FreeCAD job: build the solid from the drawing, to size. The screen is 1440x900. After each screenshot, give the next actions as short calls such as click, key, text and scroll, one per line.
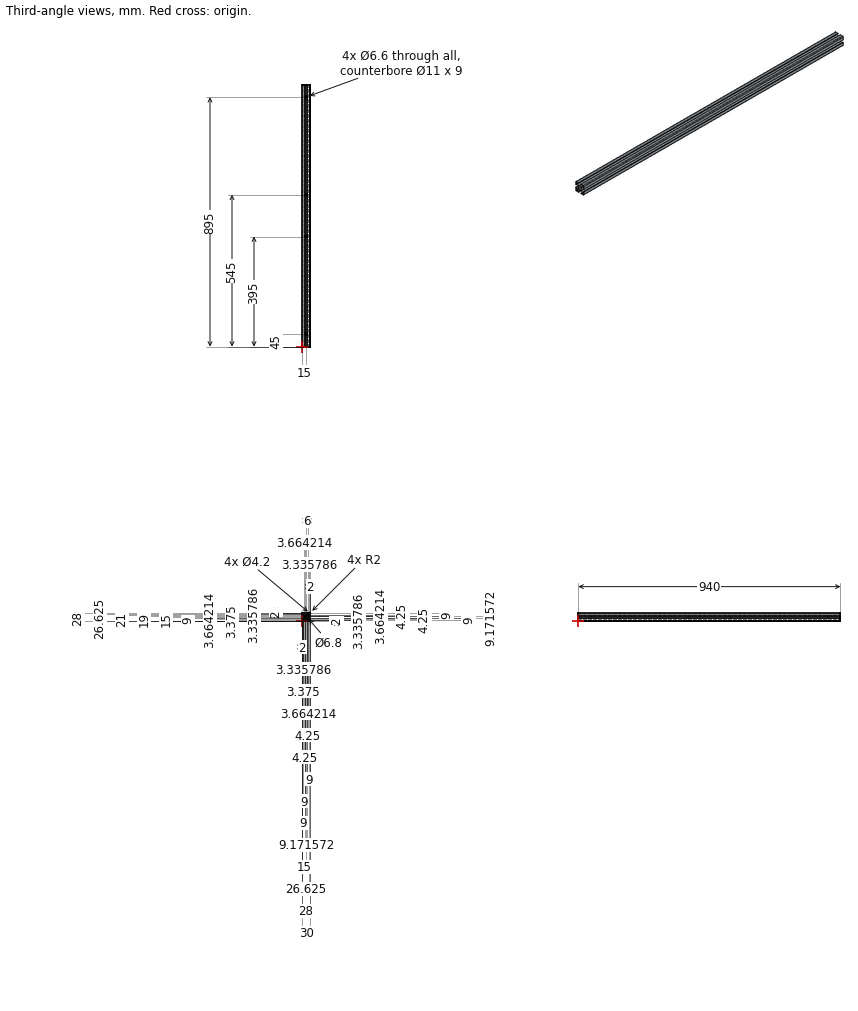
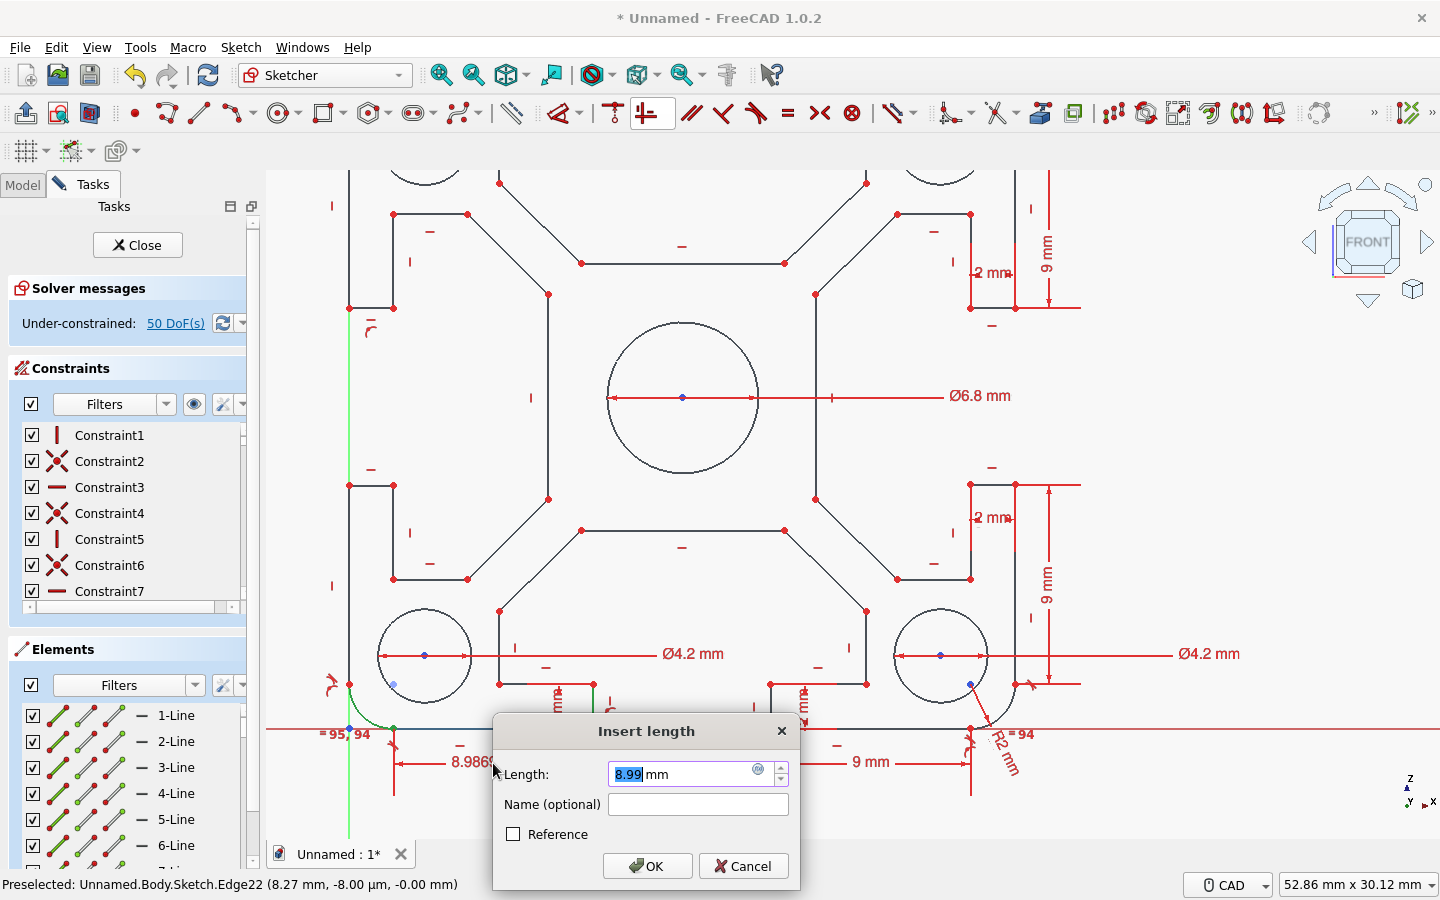
text(9)
key(Return)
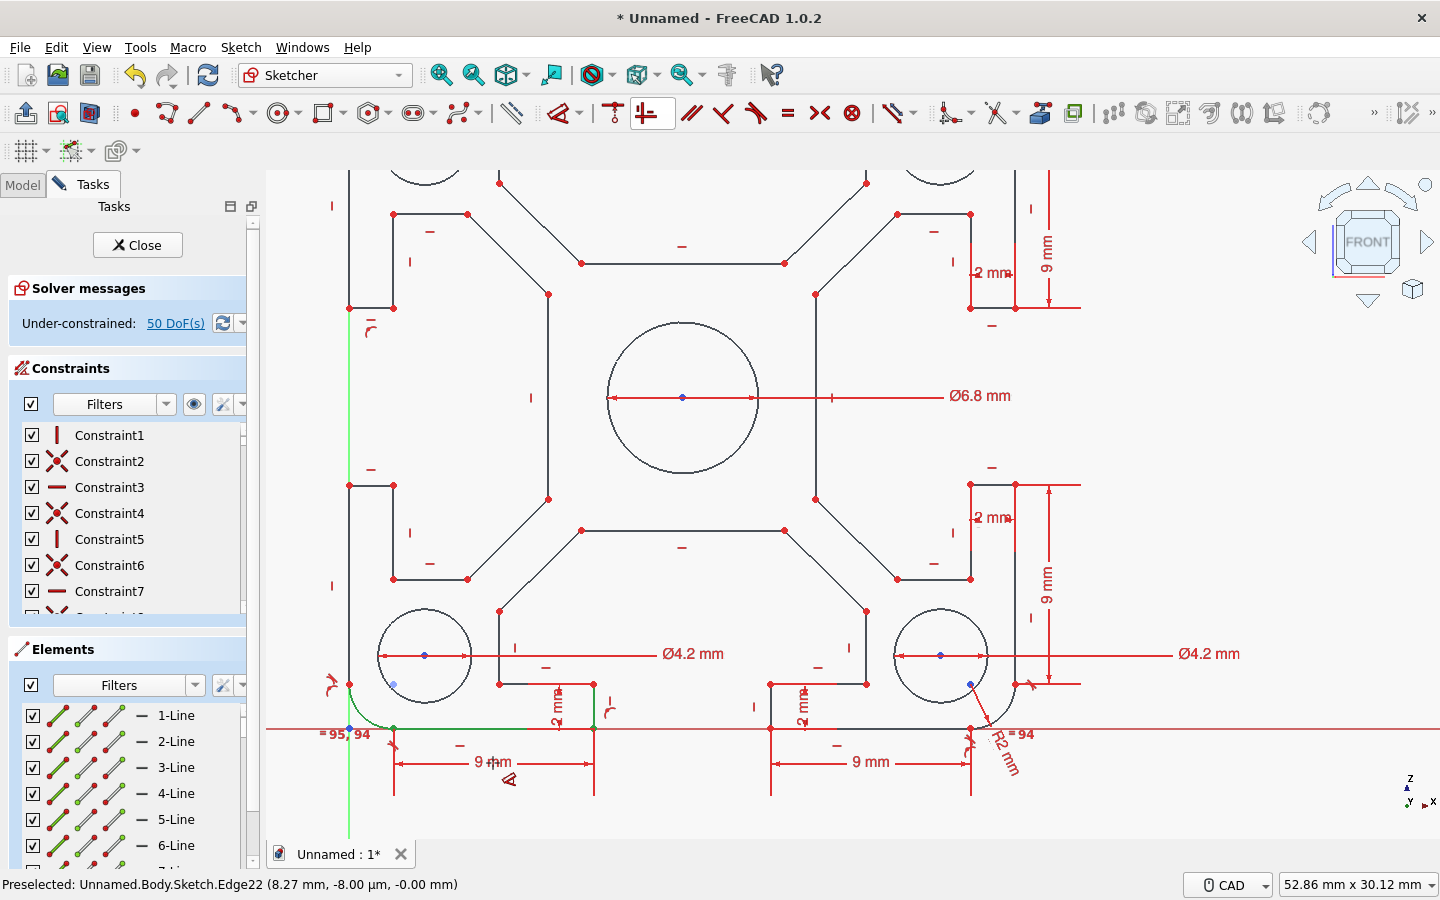
click(349, 625)
click(315, 585)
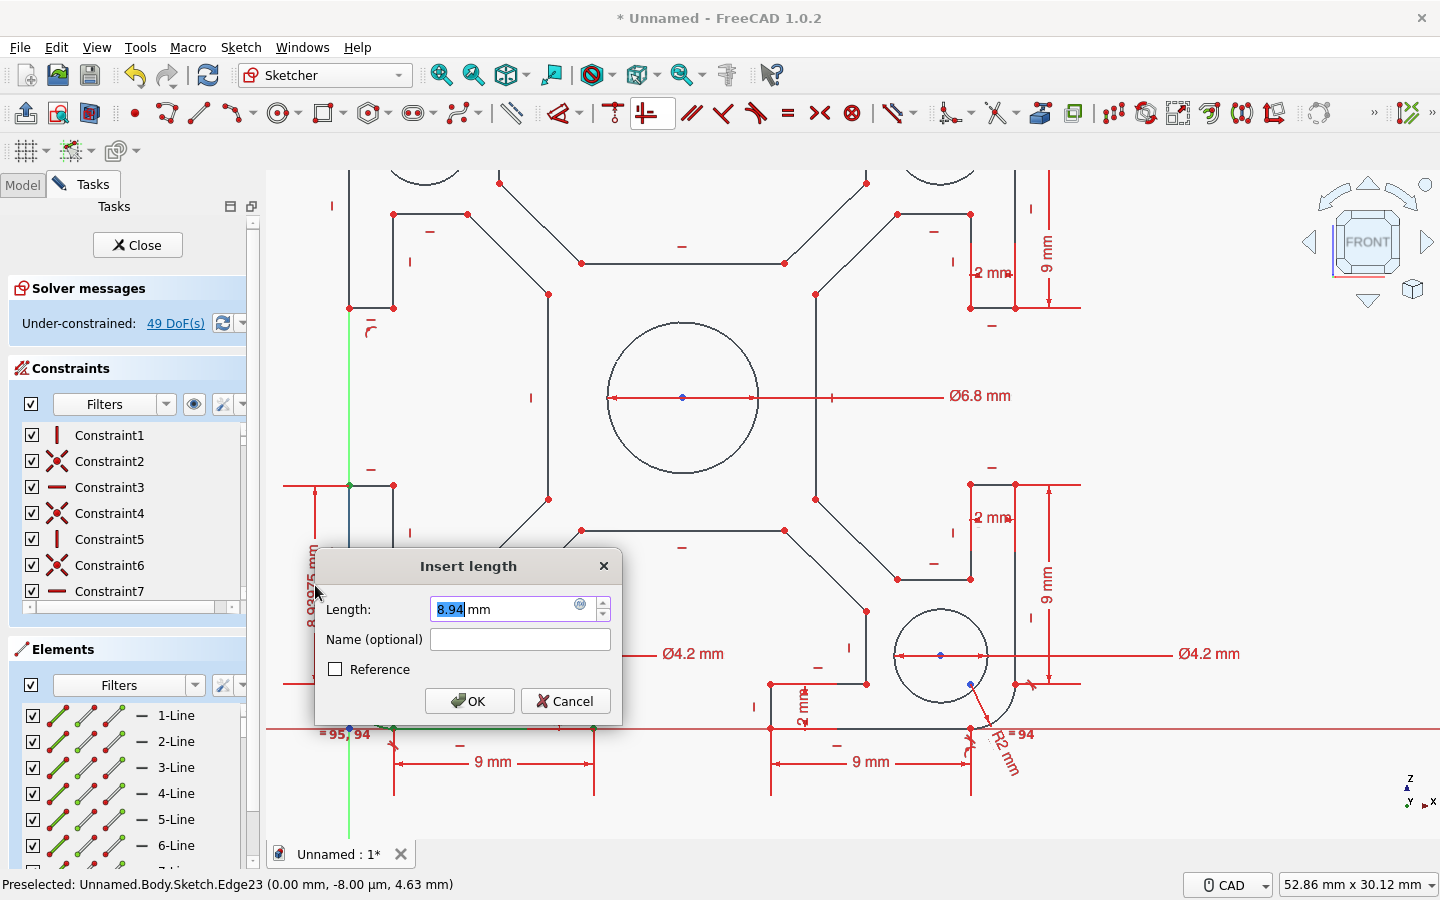
text(9)
key(Return)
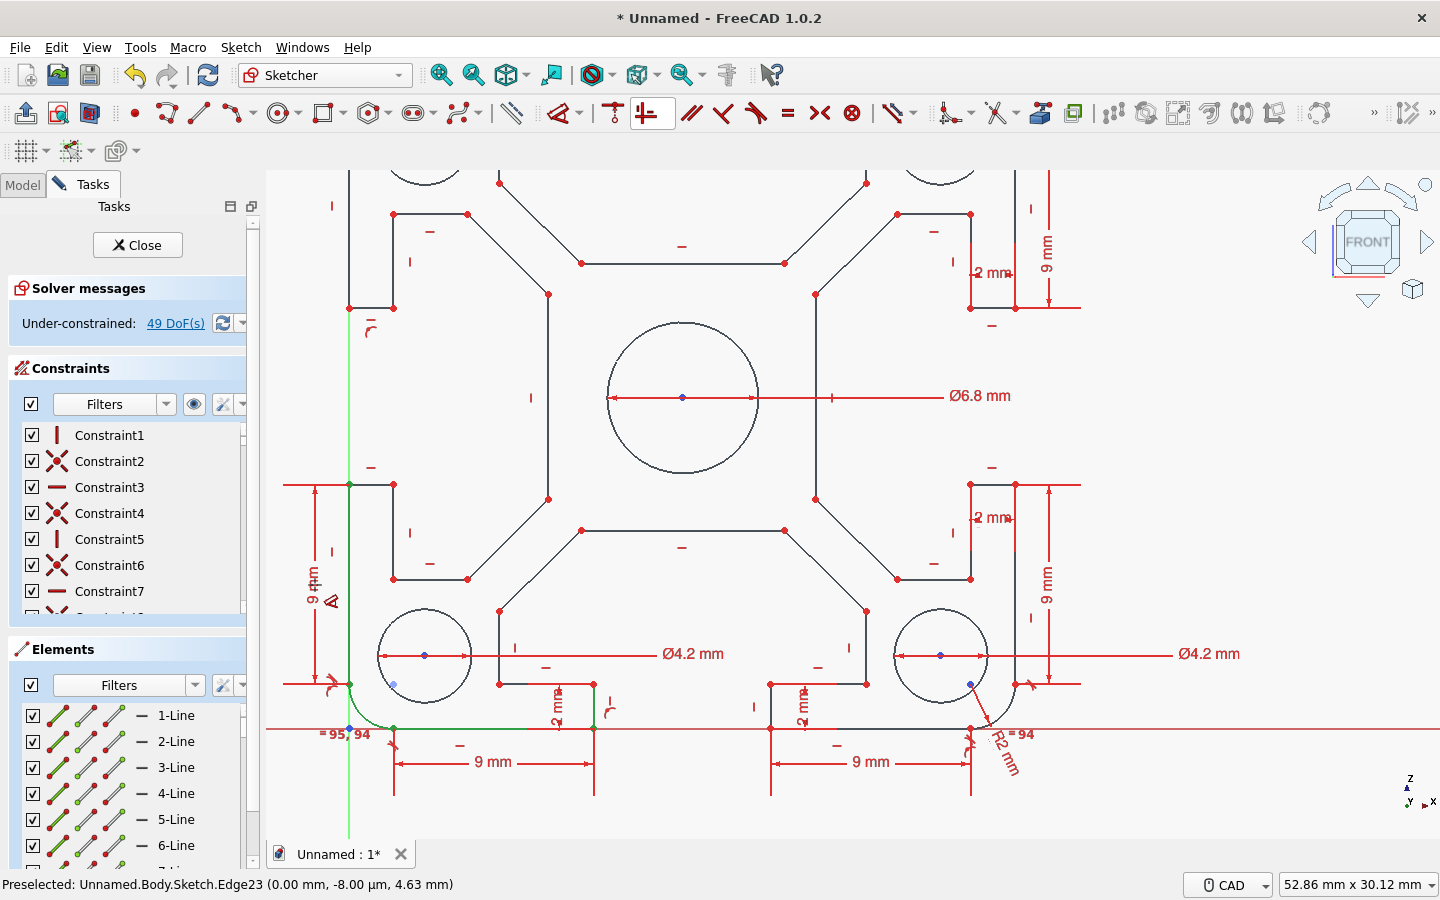
click(362, 485)
click(371, 519)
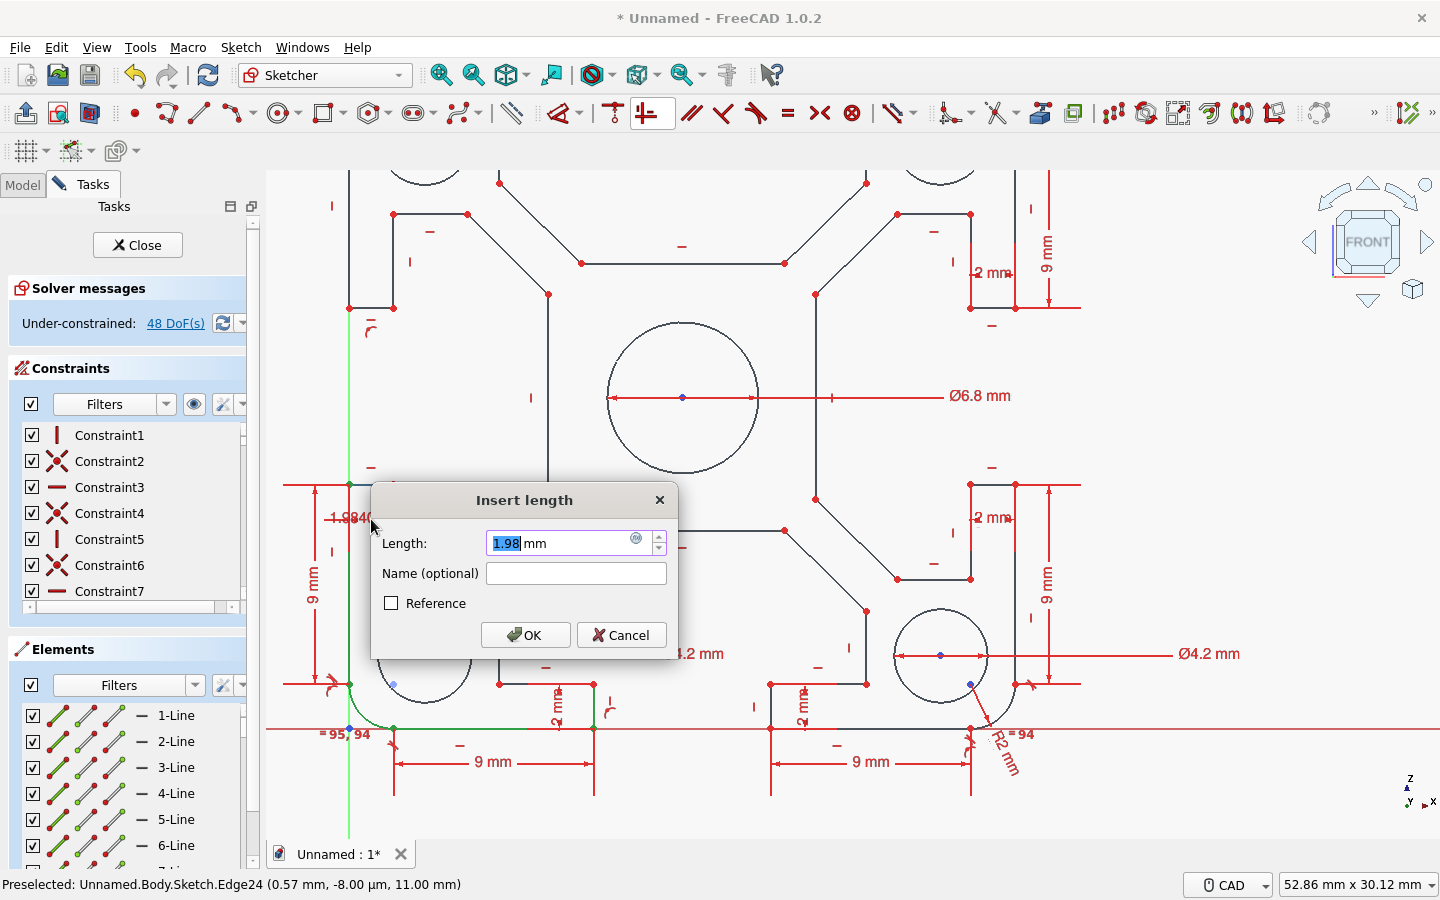
text(2)
key(Return)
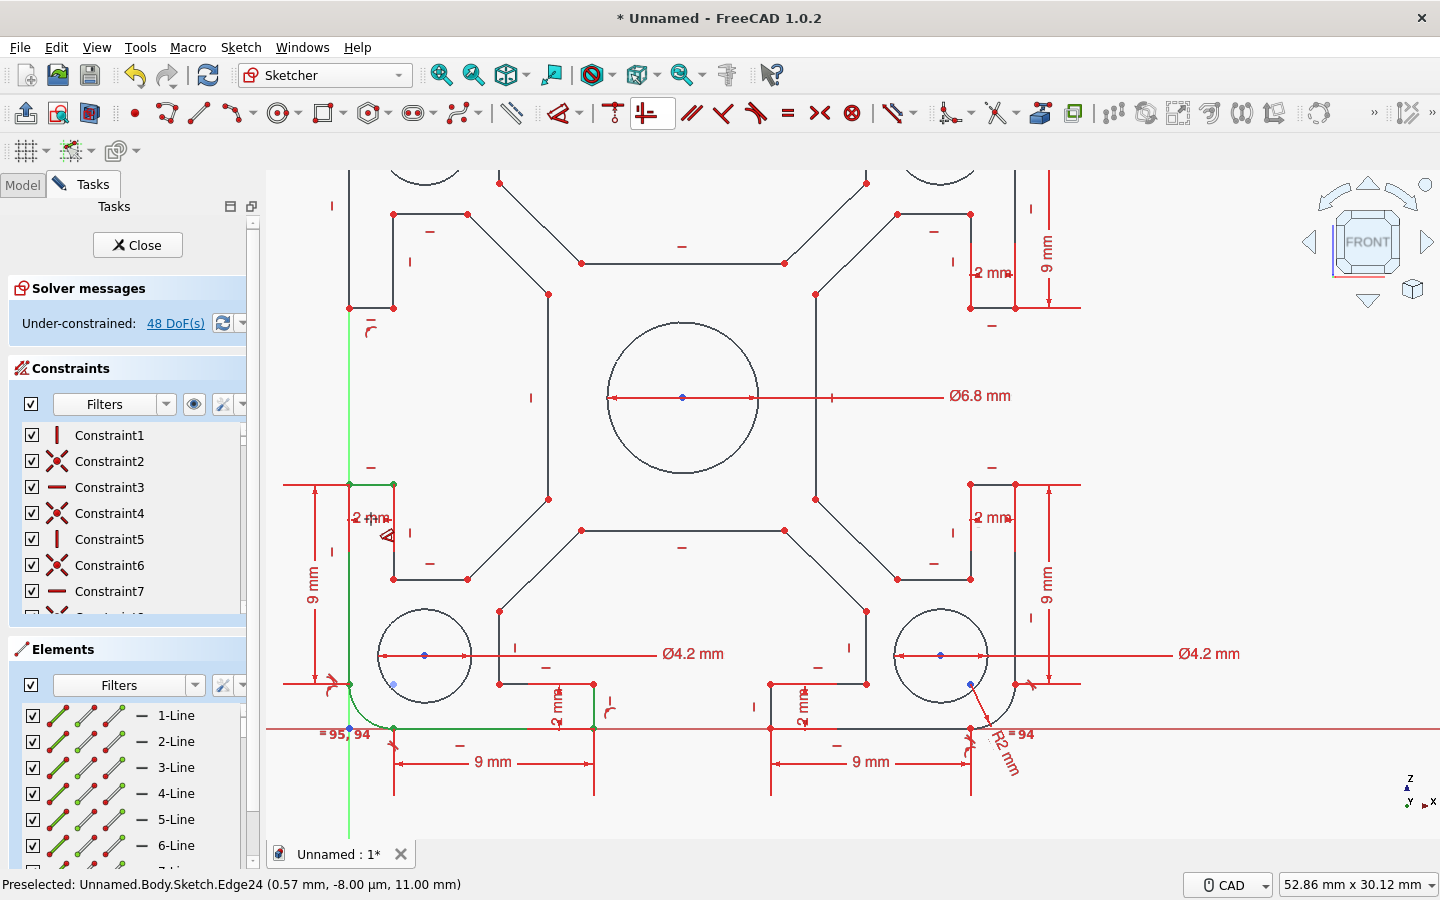
click(380, 308)
click(371, 274)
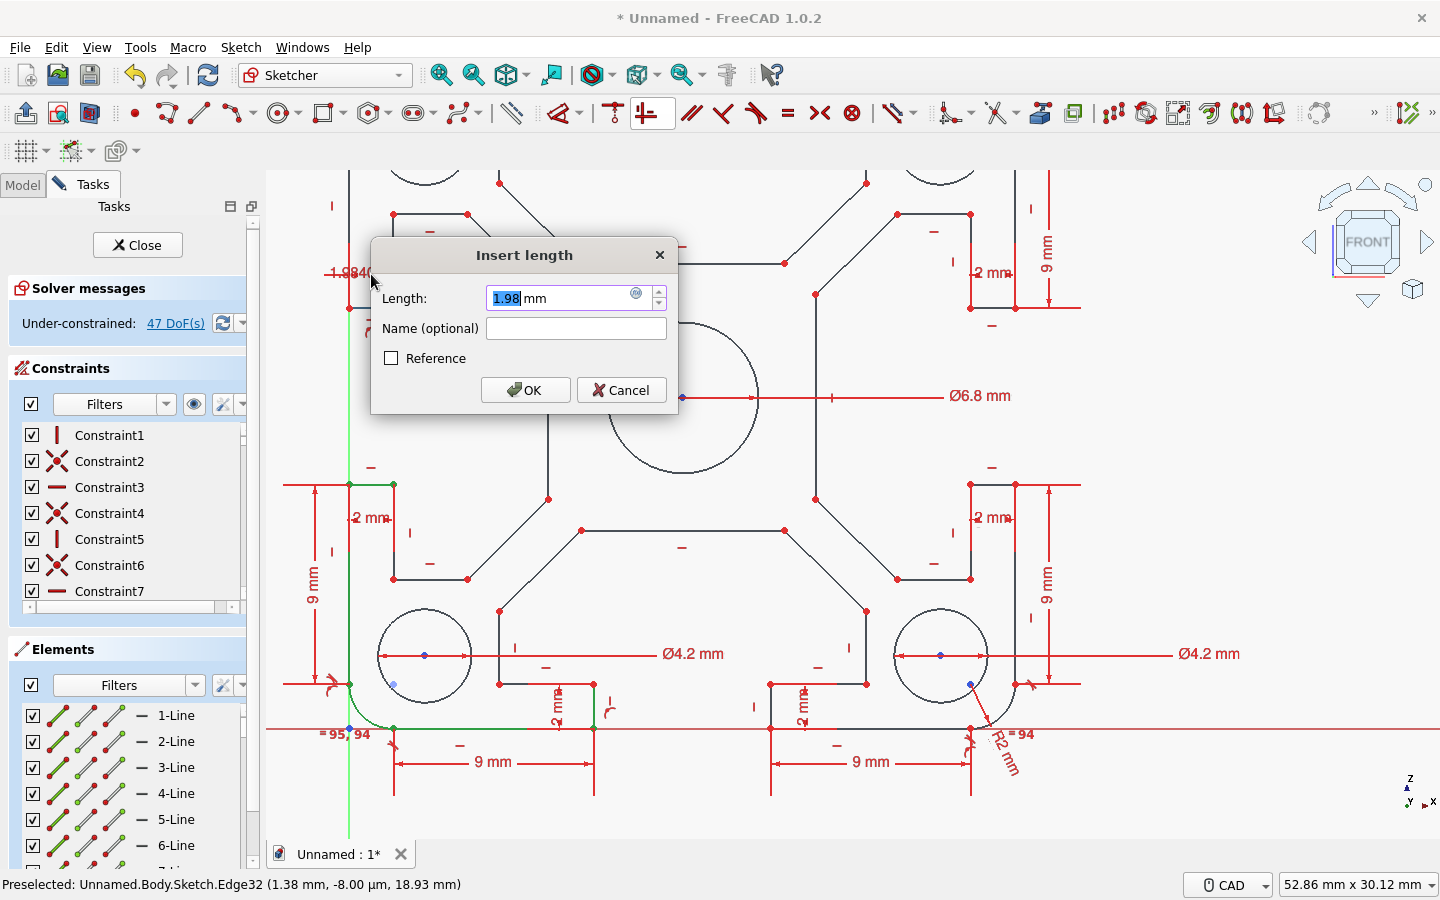
text(2)
key(Return)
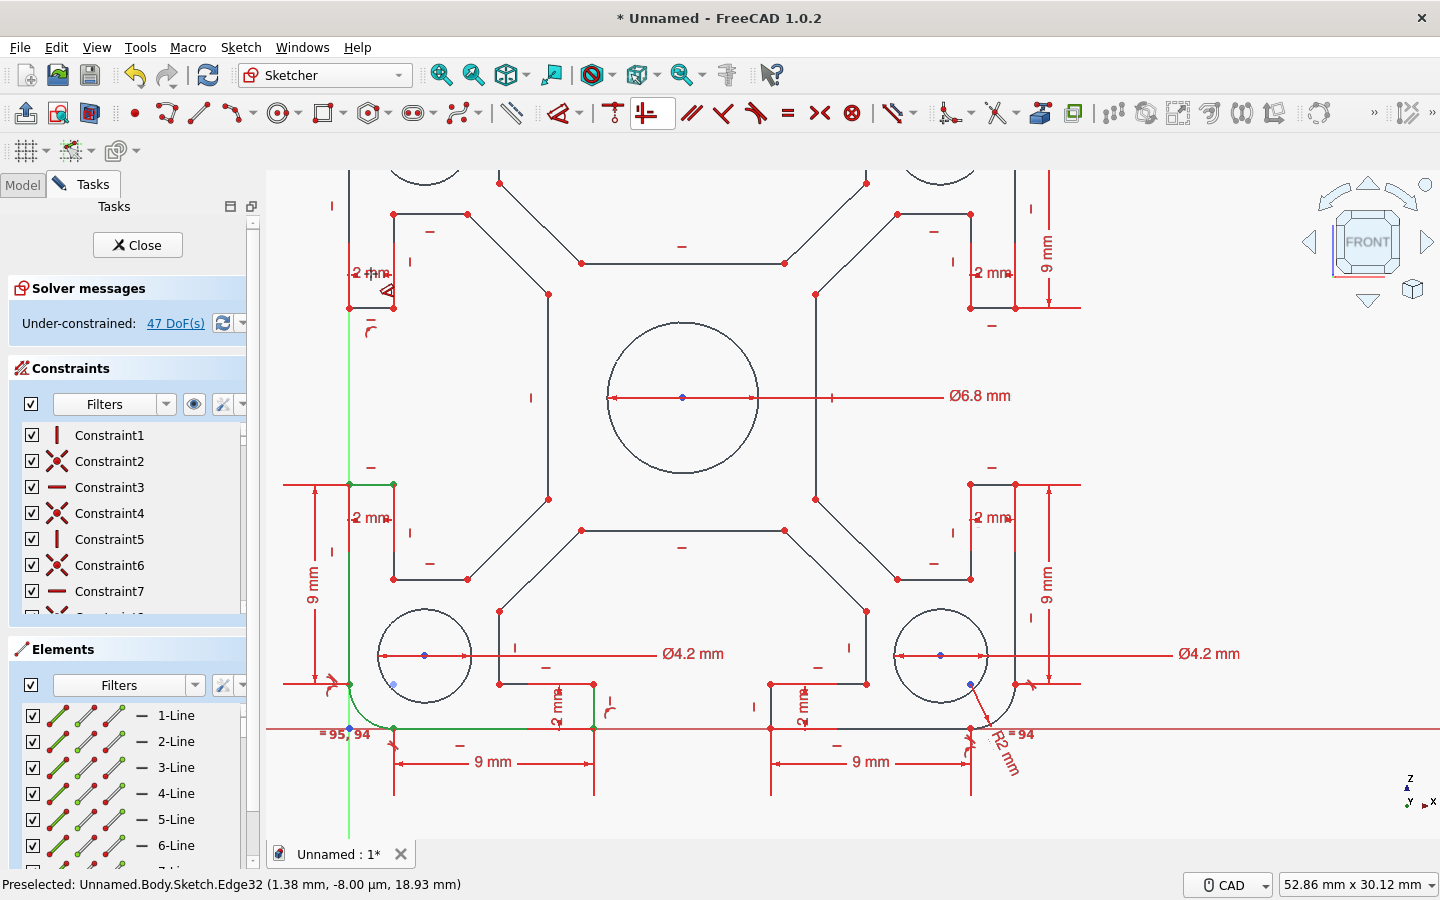
click(349, 247)
click(315, 253)